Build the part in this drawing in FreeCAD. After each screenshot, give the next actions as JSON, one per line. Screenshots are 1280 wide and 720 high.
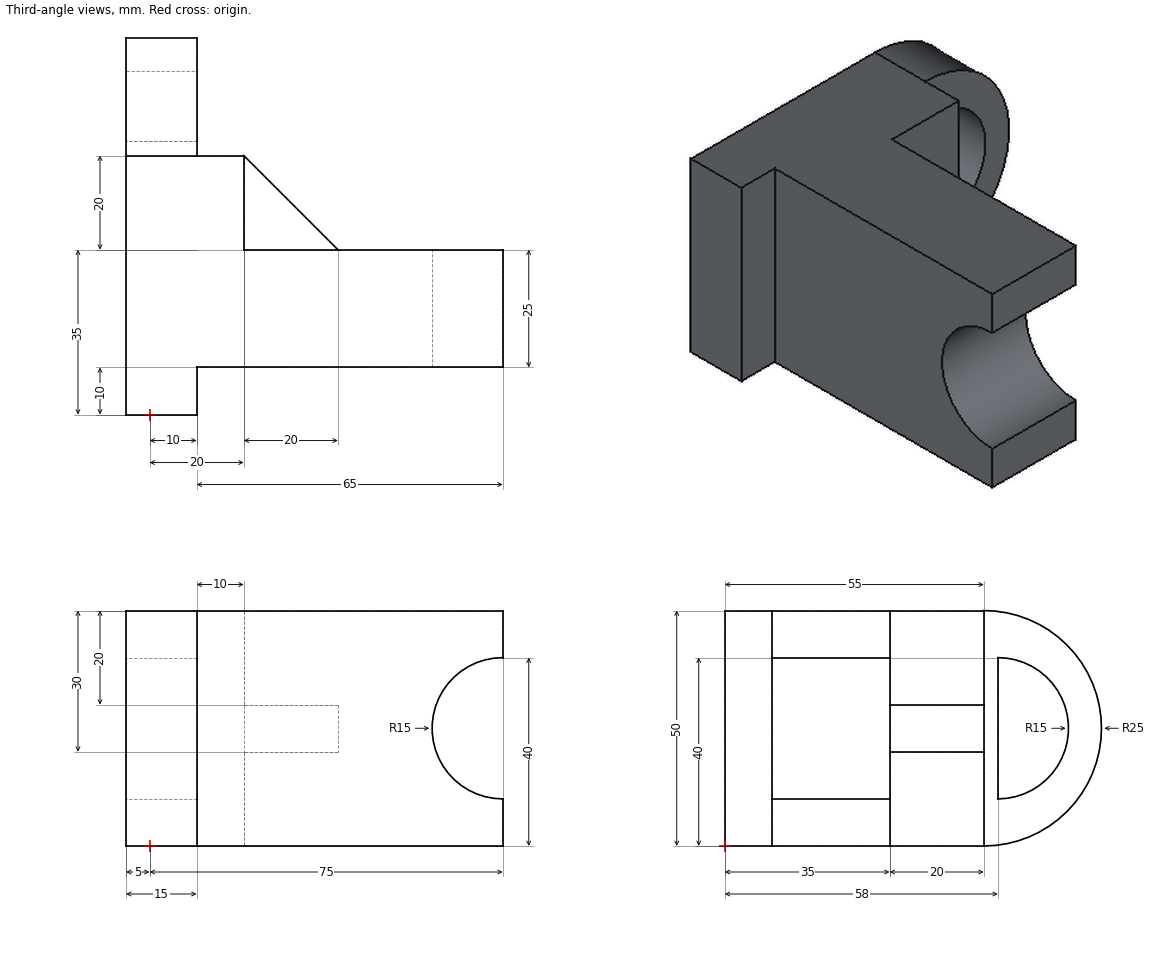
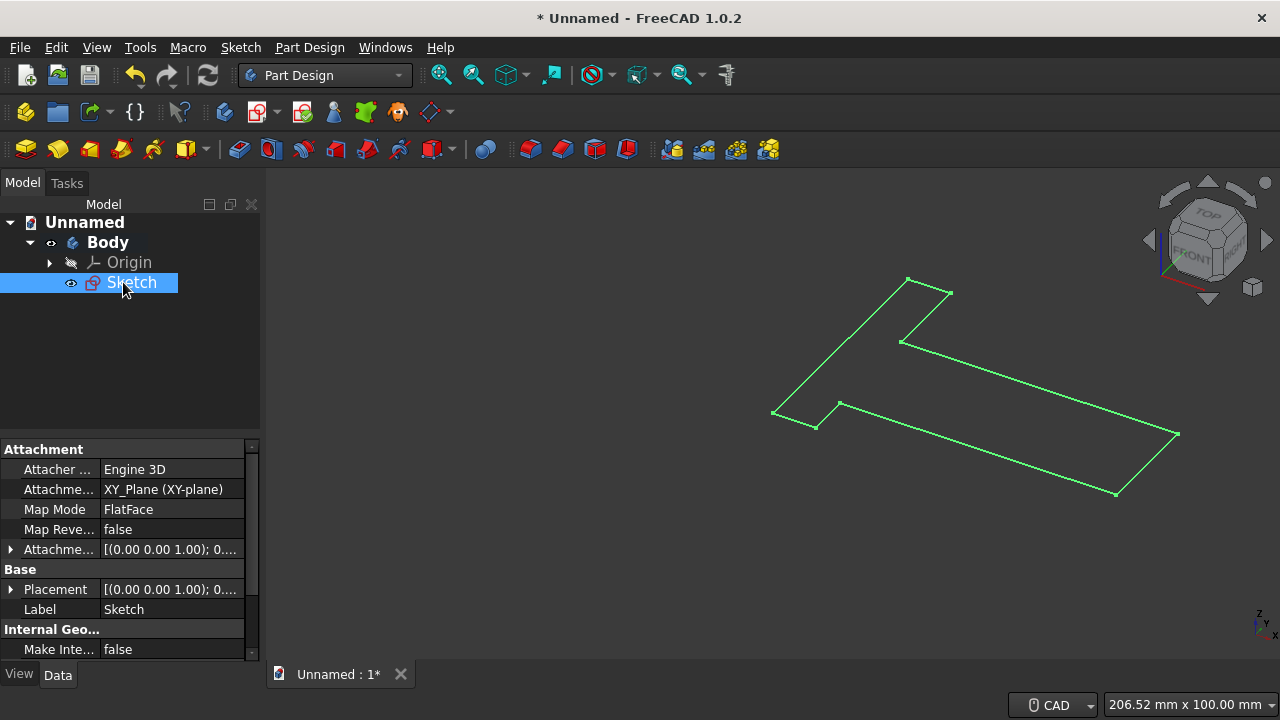
{"action": "left_click", "coordinate": [26, 150]}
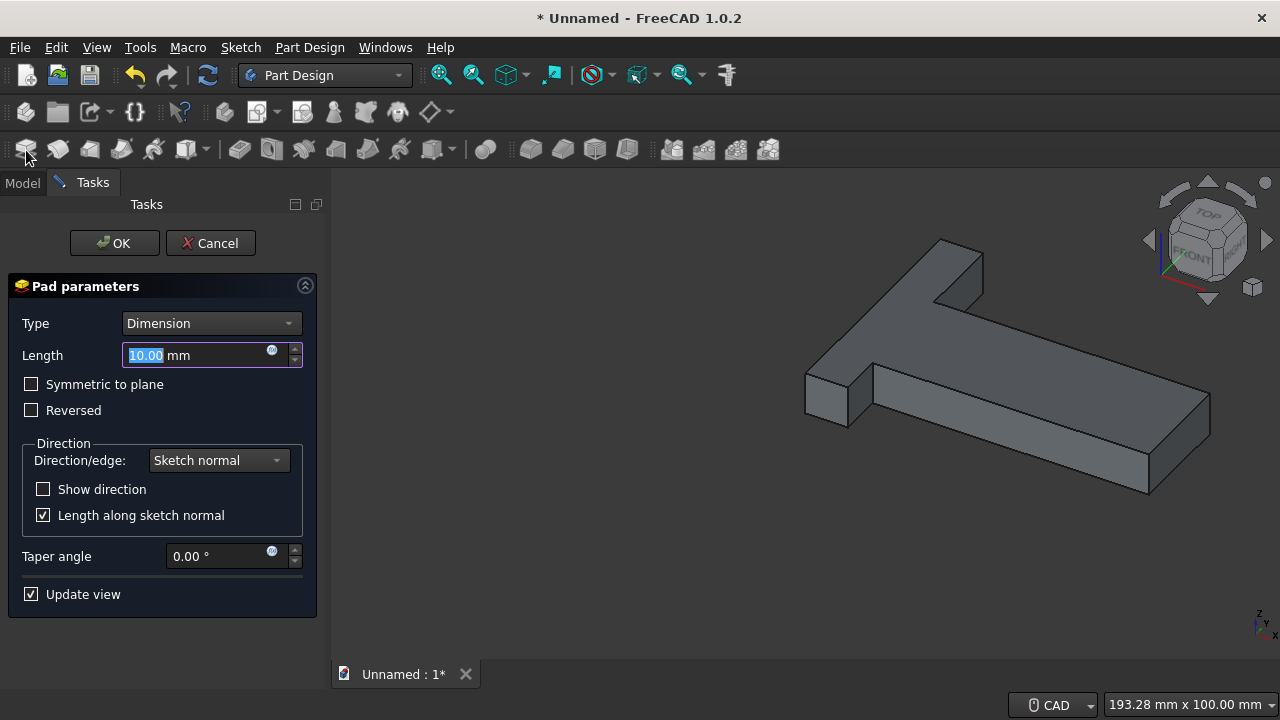
{"action": "type", "text": "50"}
{"action": "key", "text": "Tab"}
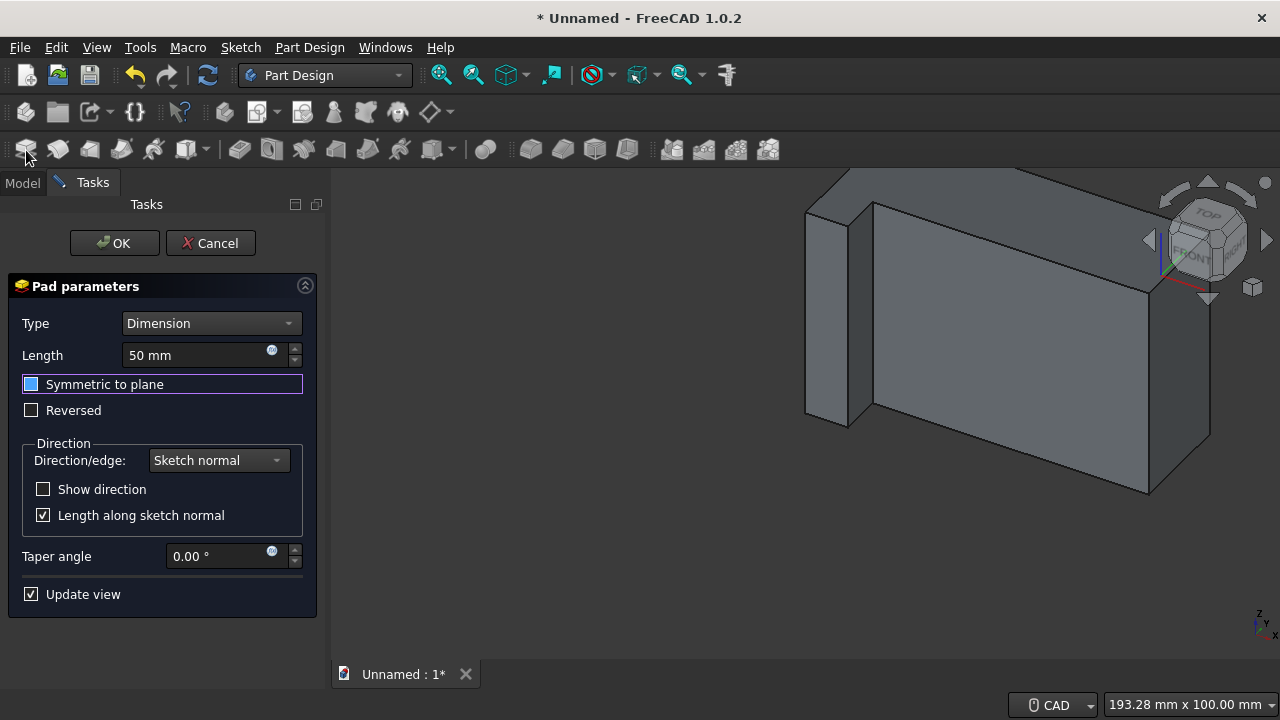
{"action": "left_click", "coordinate": [115, 243]}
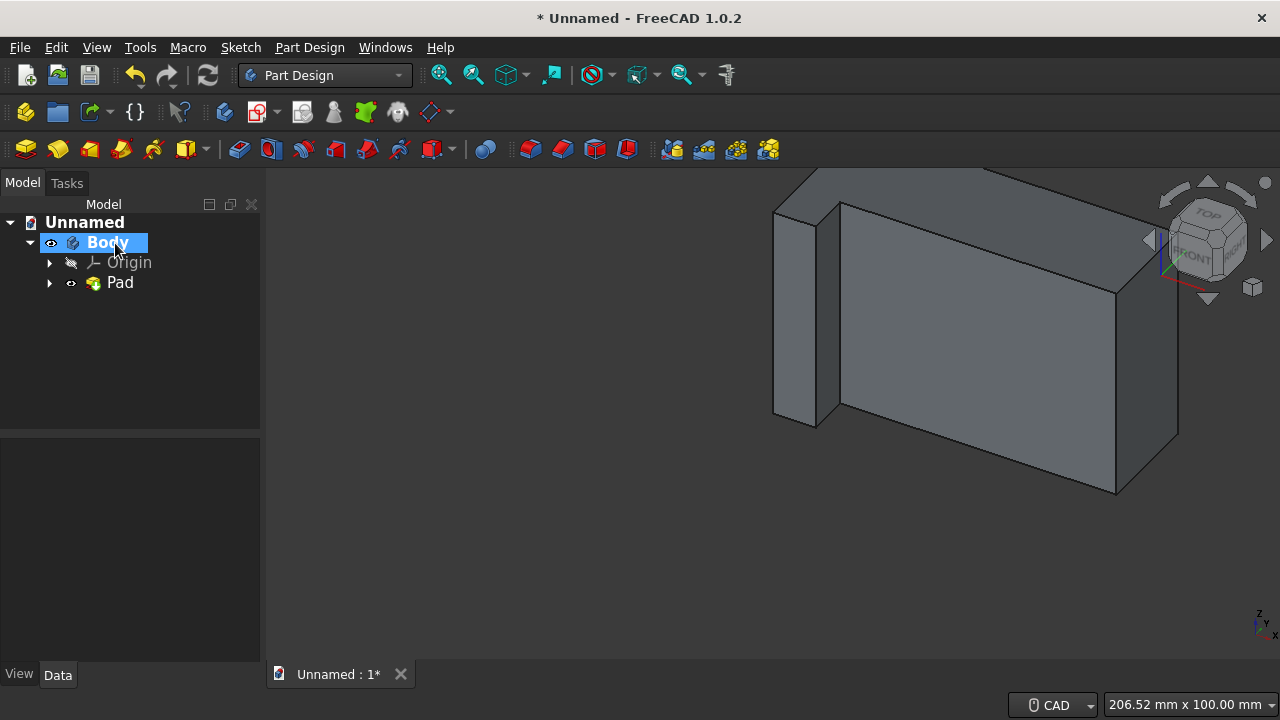
{"action": "left_click", "coordinate": [442, 76]}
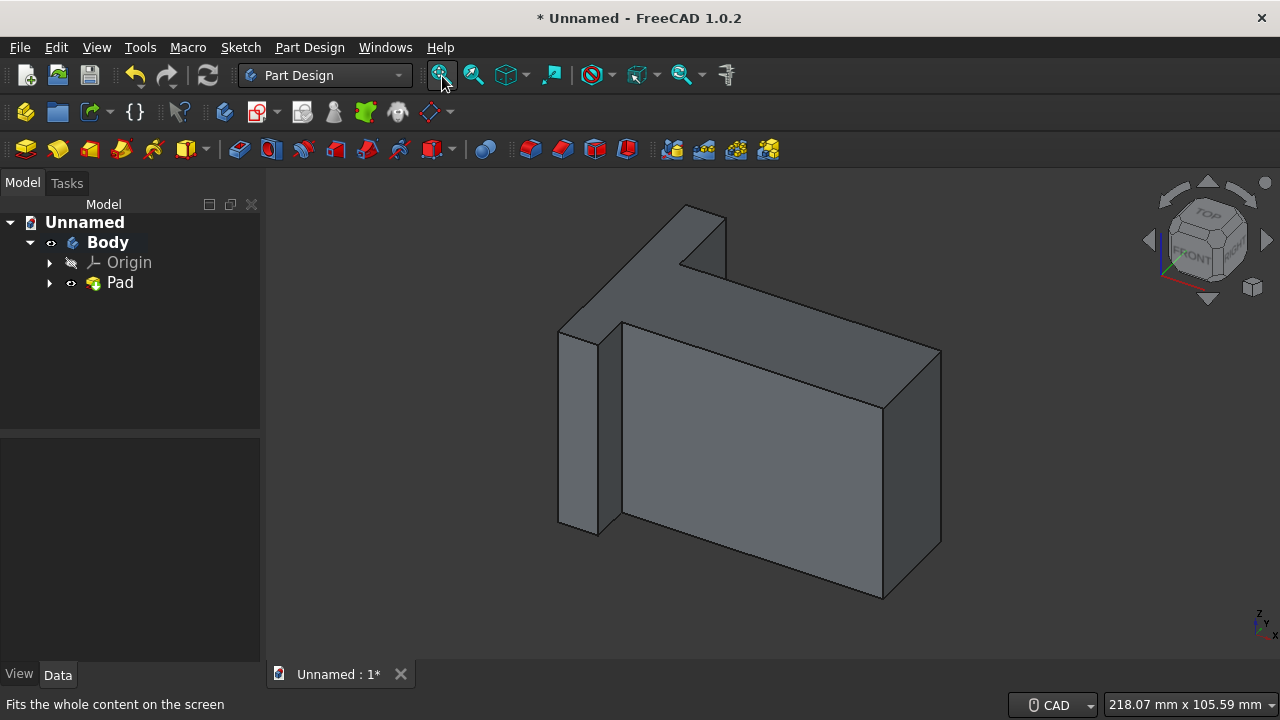
{"action": "key", "text": "6"}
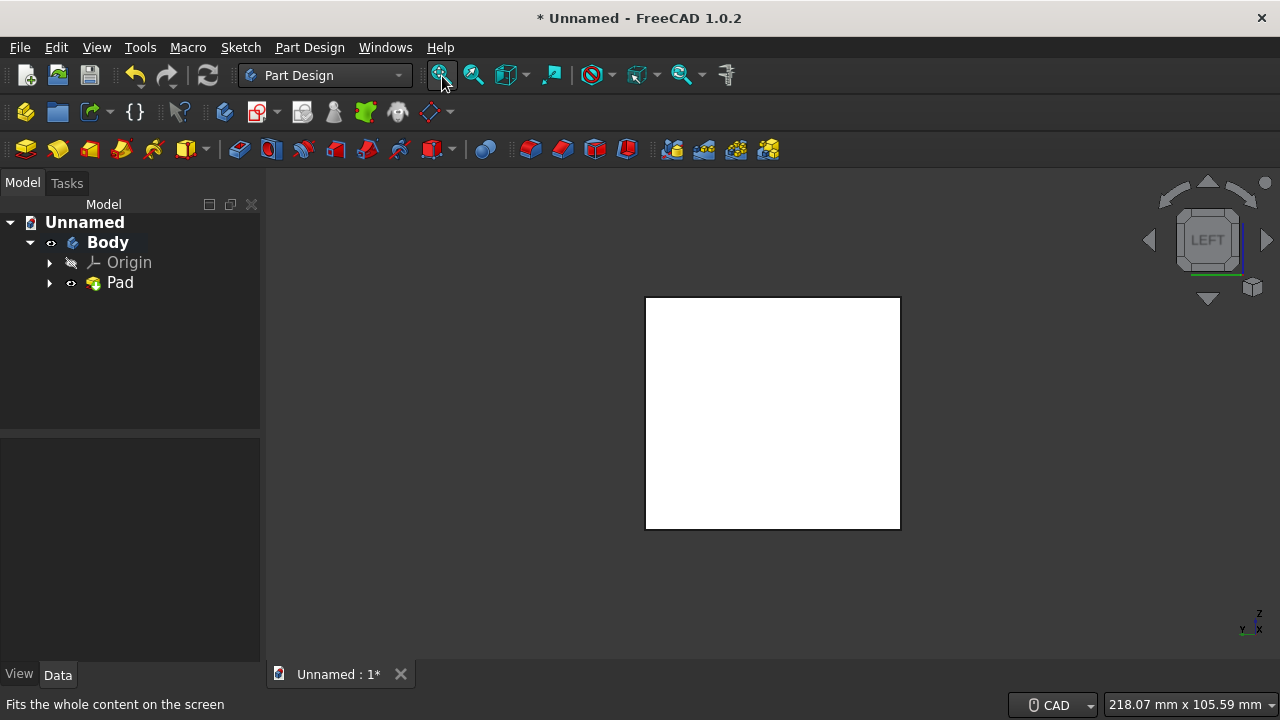
{"action": "left_click", "coordinate": [773, 413]}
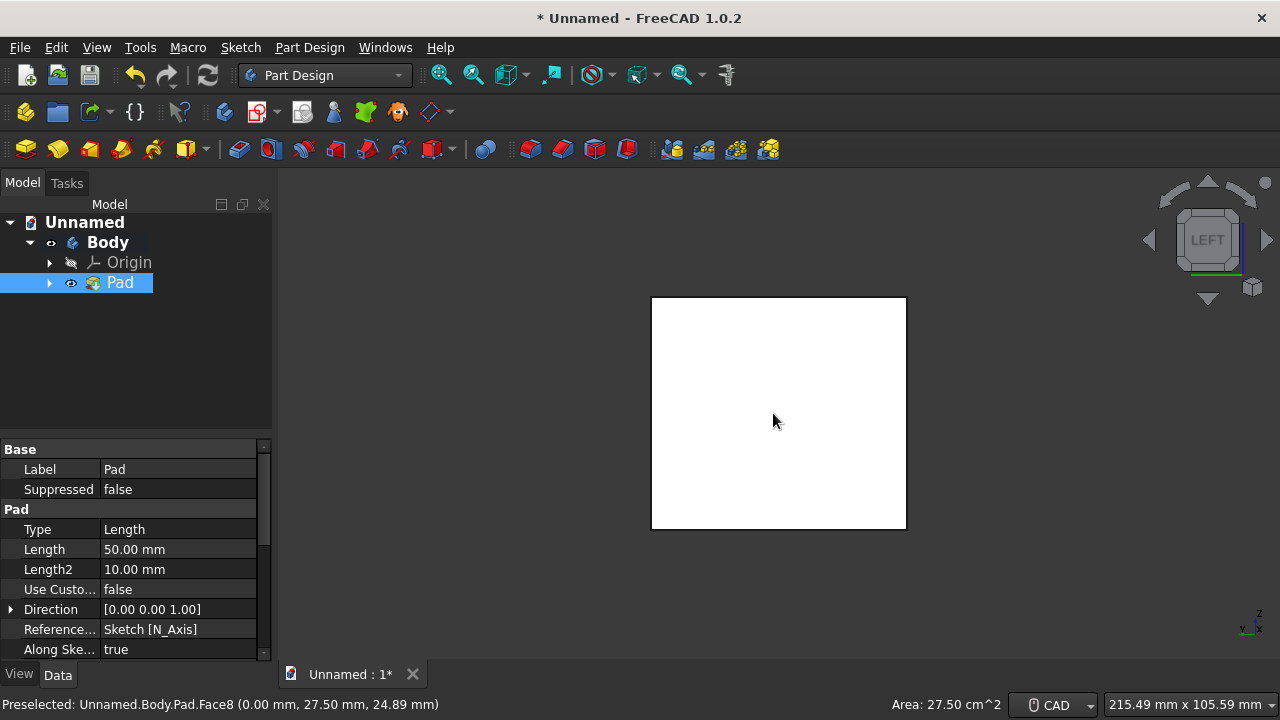
{"action": "left_click", "coordinate": [258, 112]}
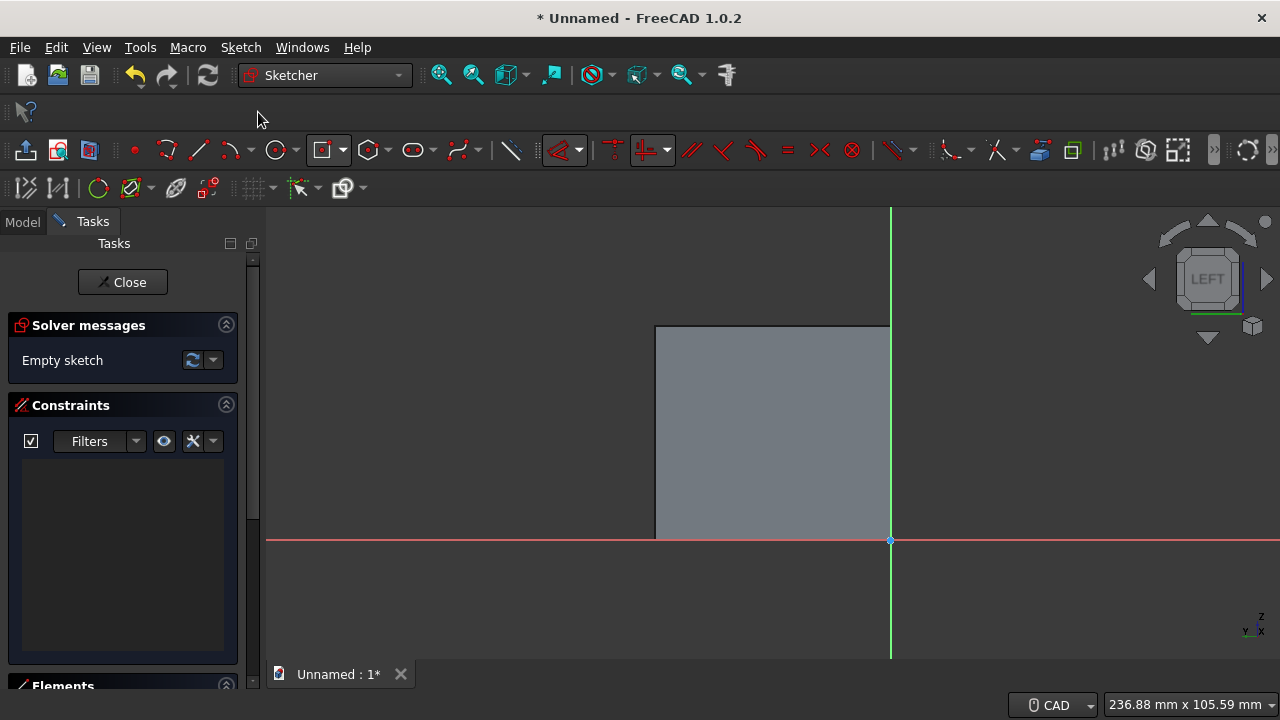
{"action": "key", "text": "g r"}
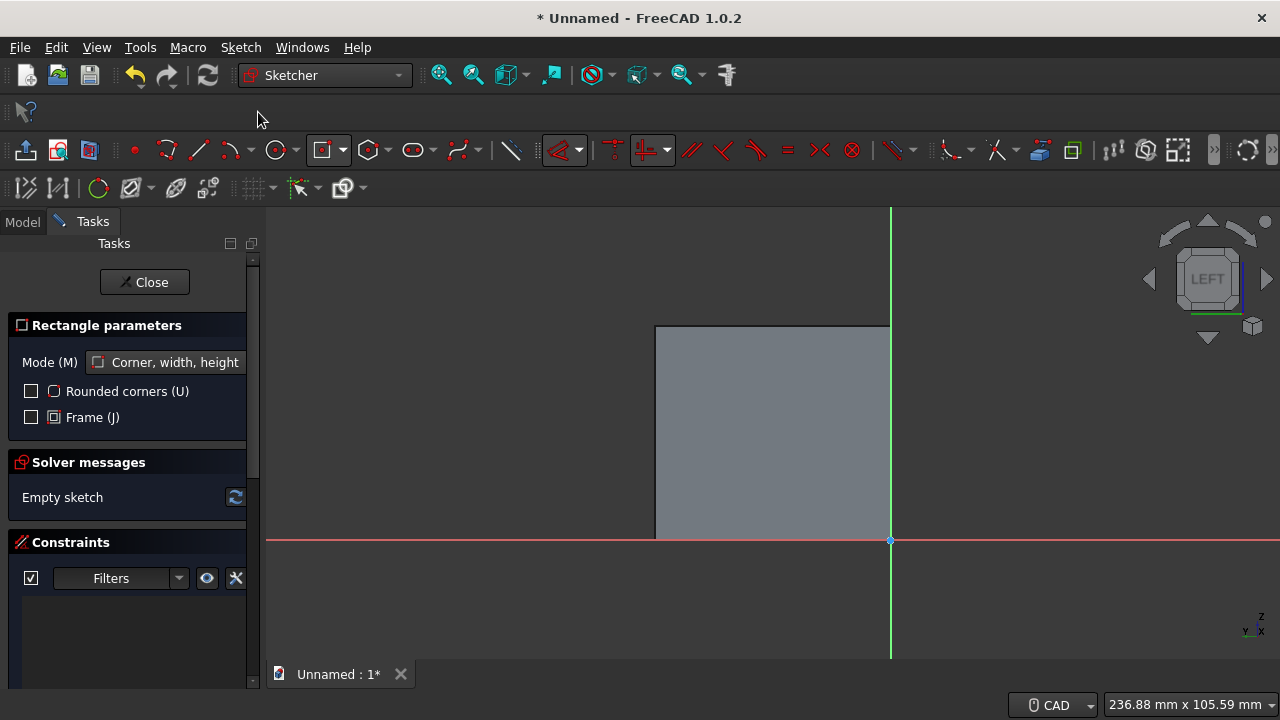
{"action": "left_click", "coordinate": [891, 540]}
{"action": "left_click", "coordinate": [655, 326]}
{"action": "key", "text": "Escape"}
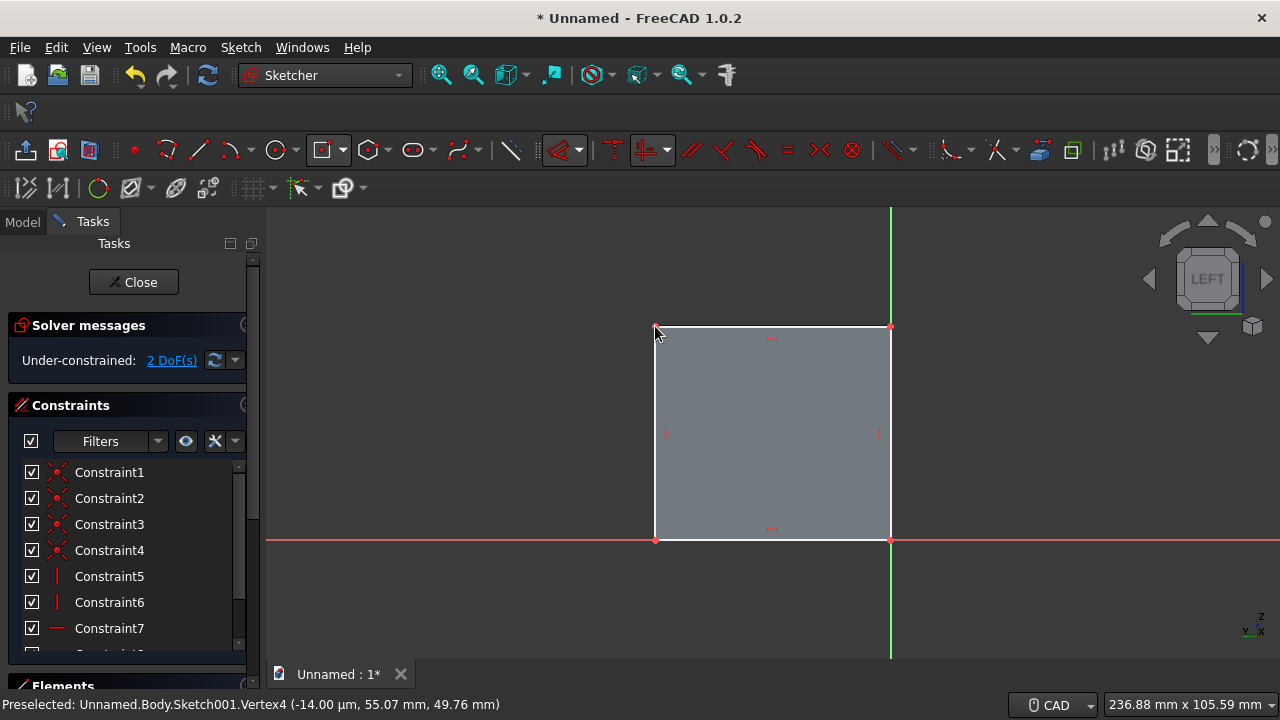
{"action": "left_click", "coordinate": [891, 476]}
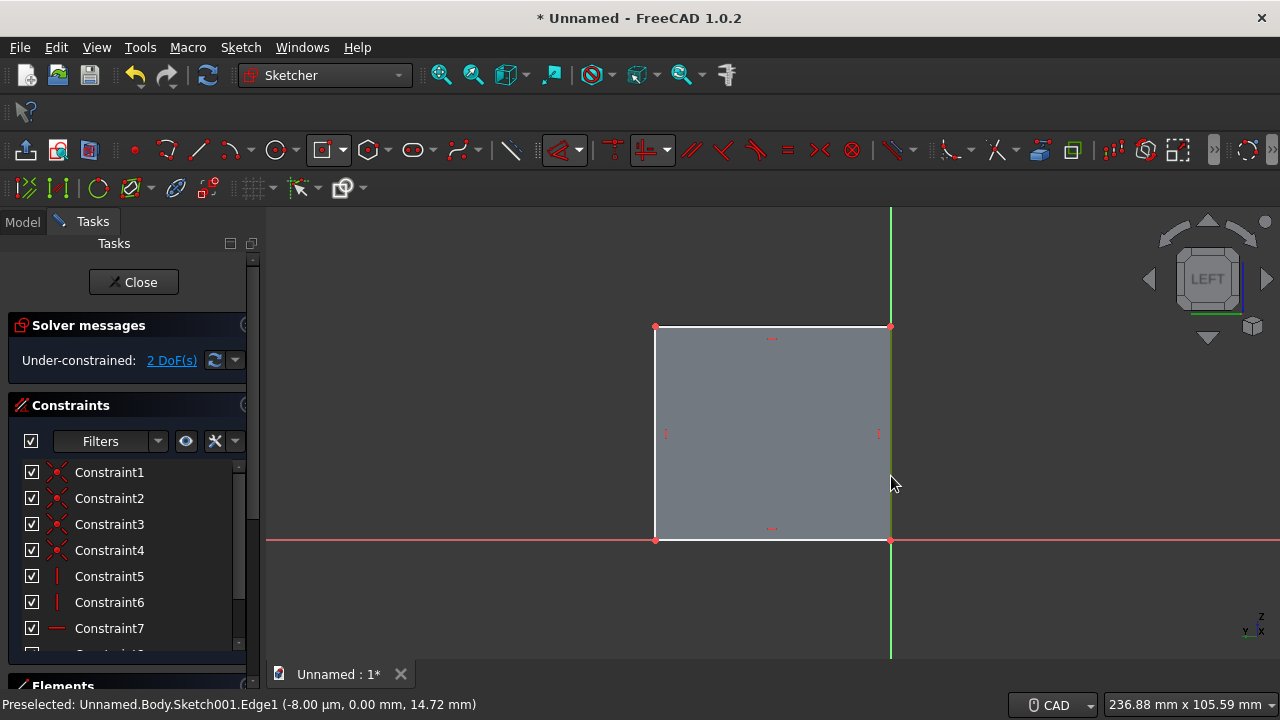
{"action": "left_click", "coordinate": [582, 150]}